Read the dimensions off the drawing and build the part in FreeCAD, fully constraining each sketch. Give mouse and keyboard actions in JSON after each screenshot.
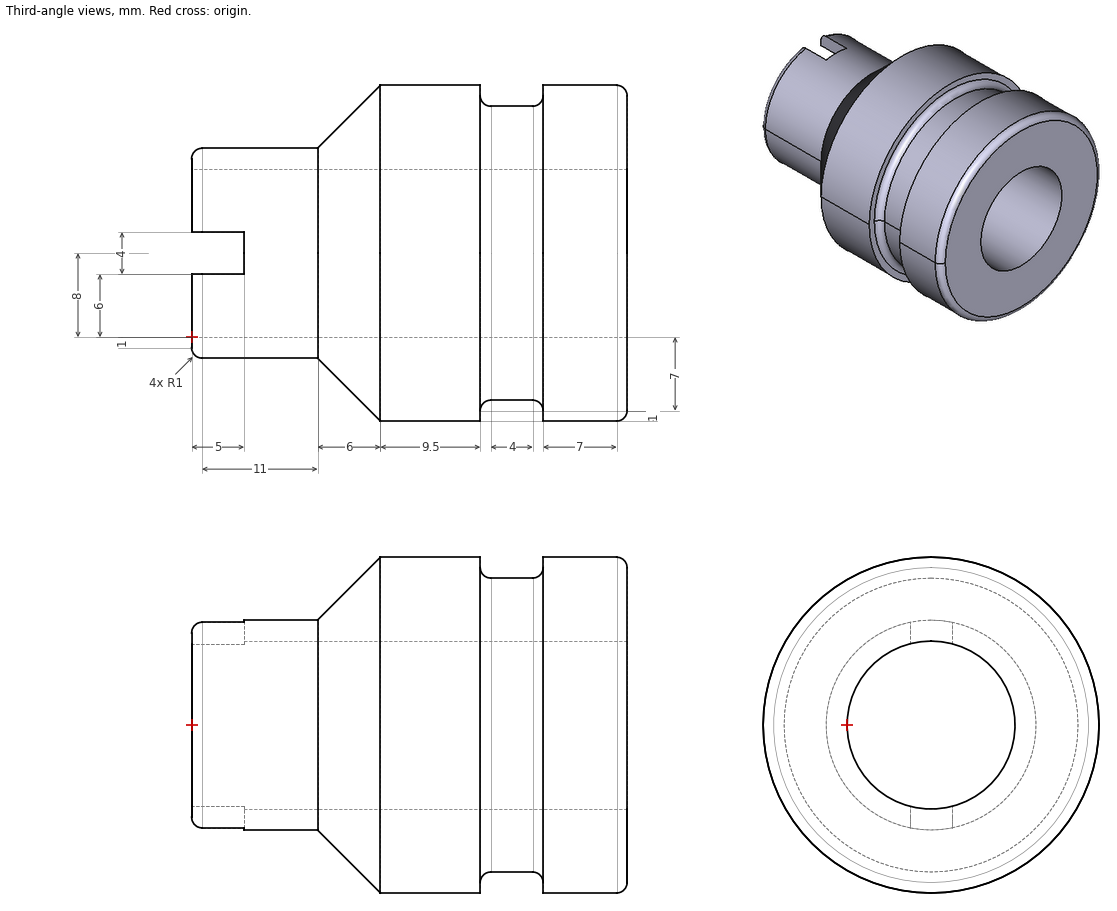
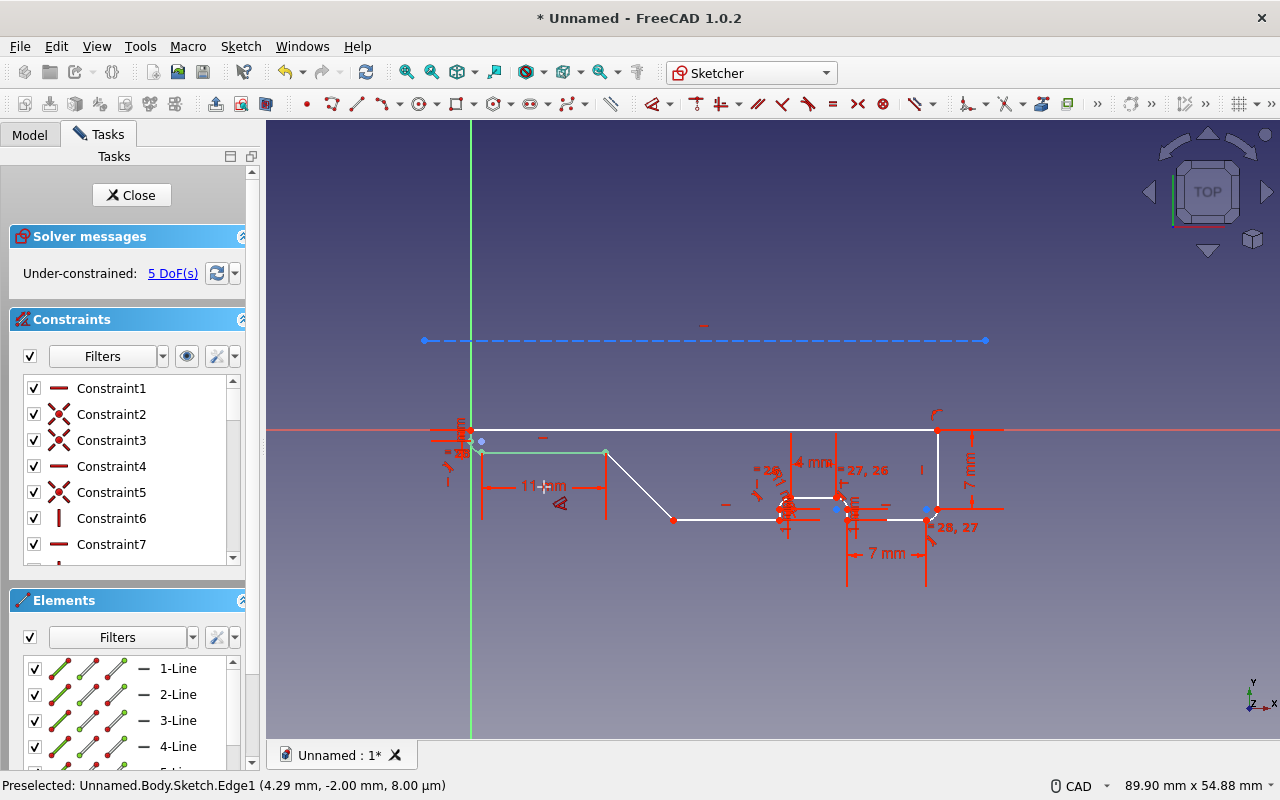
{"action": "left_click", "coordinate": [424, 341]}
{"action": "left_click", "coordinate": [390, 385]}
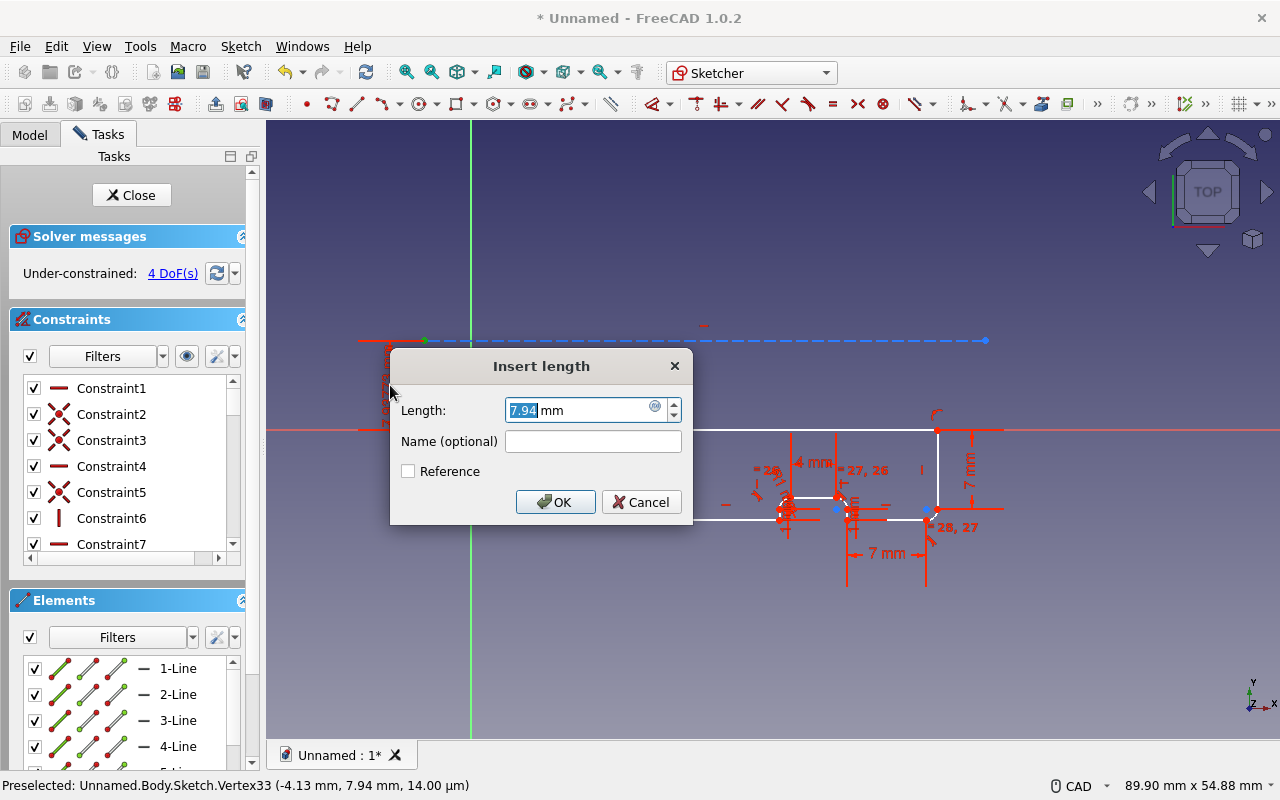
{"action": "type", "text": "8"}
{"action": "key", "text": "Return"}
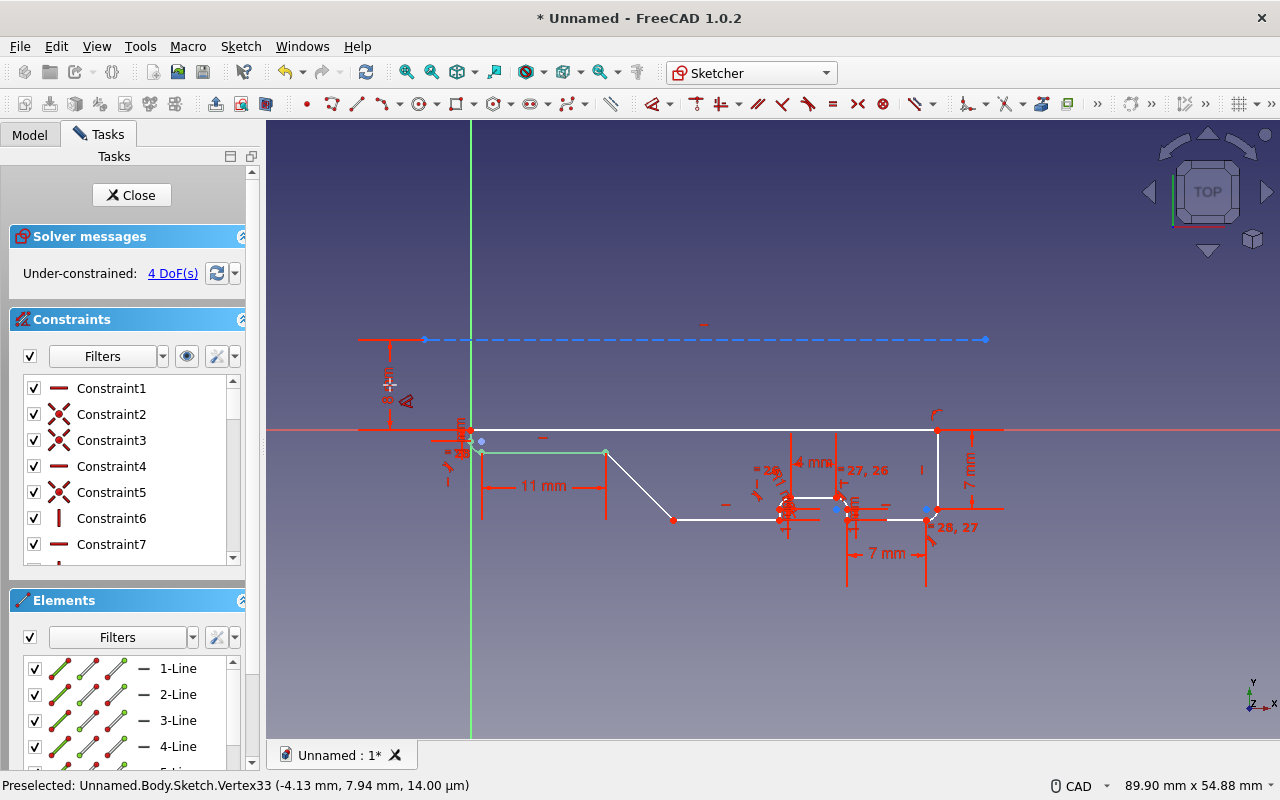
{"action": "left_click", "coordinate": [626, 473]}
{"action": "left_click", "coordinate": [640, 554]}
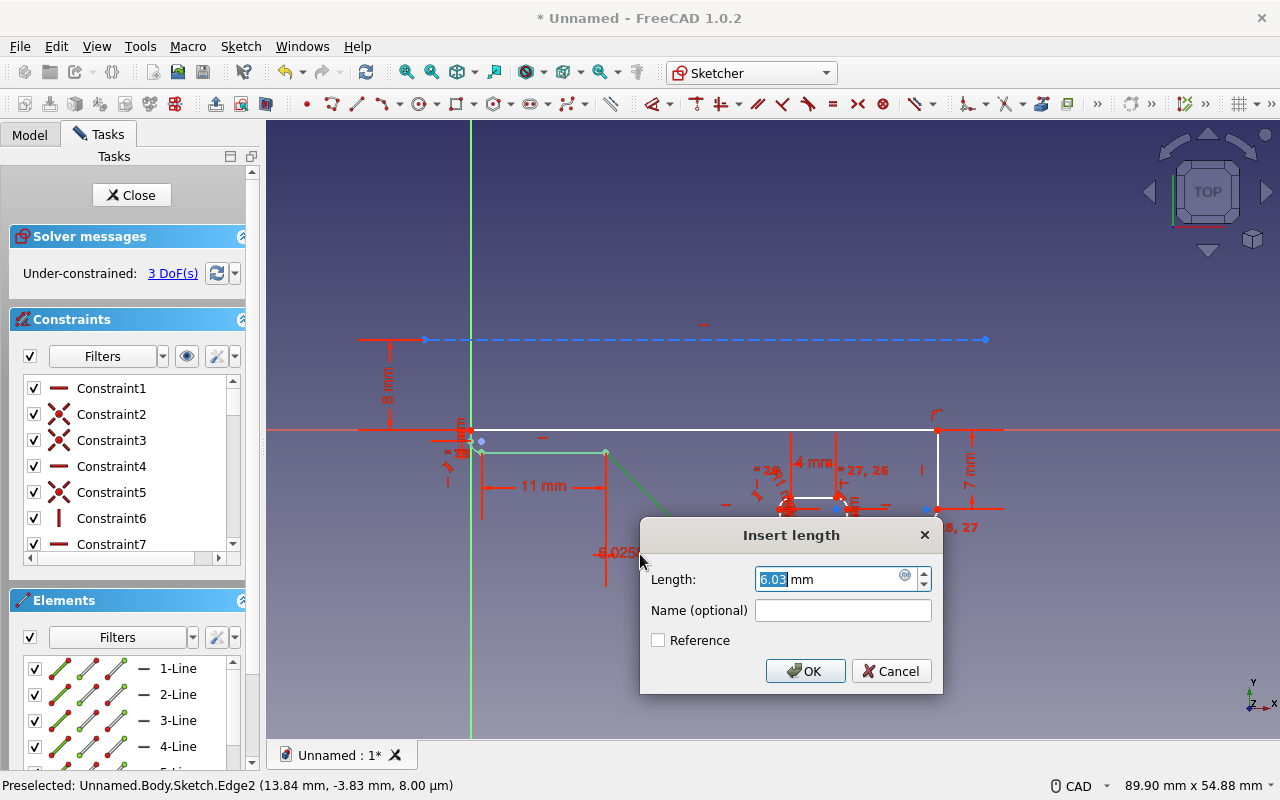
{"action": "type", "text": "6"}
{"action": "key", "text": "Return"}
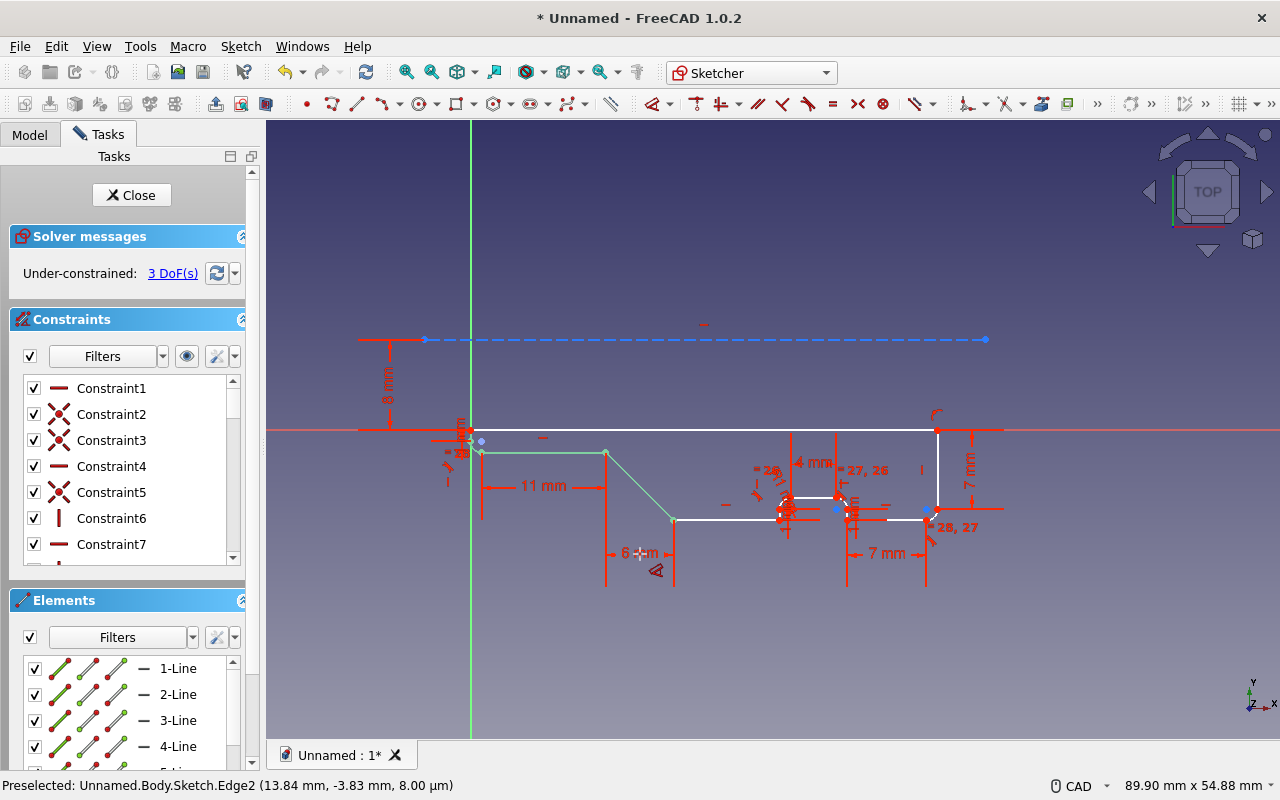
{"action": "left_click", "coordinate": [705, 520]}
{"action": "left_click", "coordinate": [727, 554]}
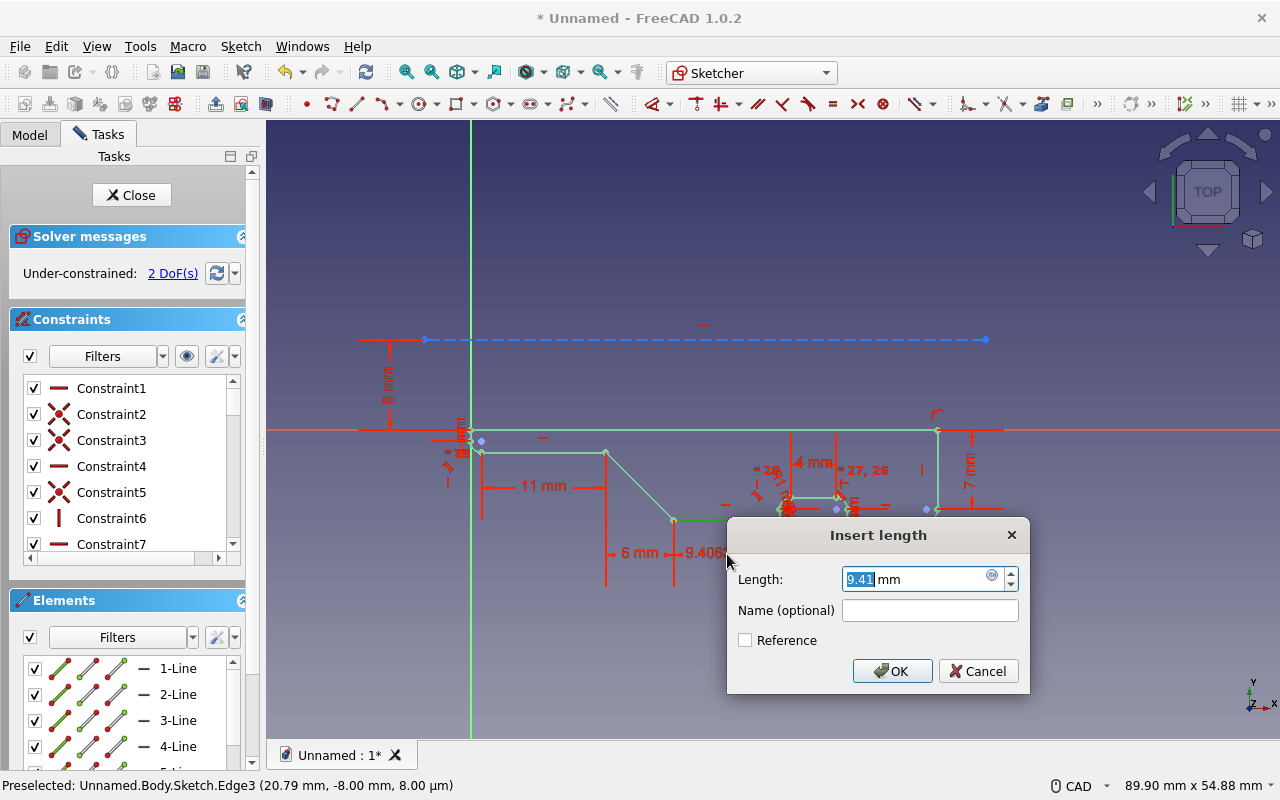
{"action": "type", "text": "9.5"}
{"action": "key", "text": "Return"}
{"action": "key", "text": "Escape"}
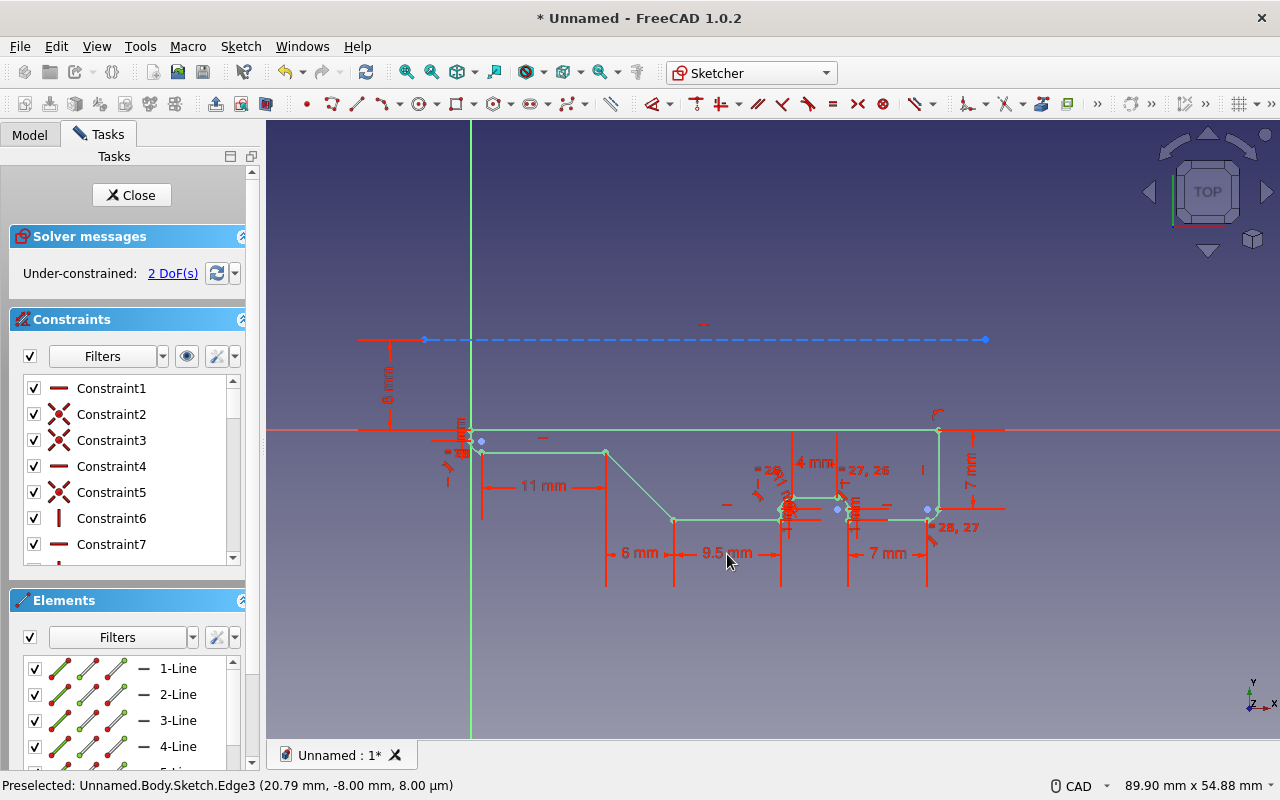
{"action": "left_click", "coordinate": [132, 195]}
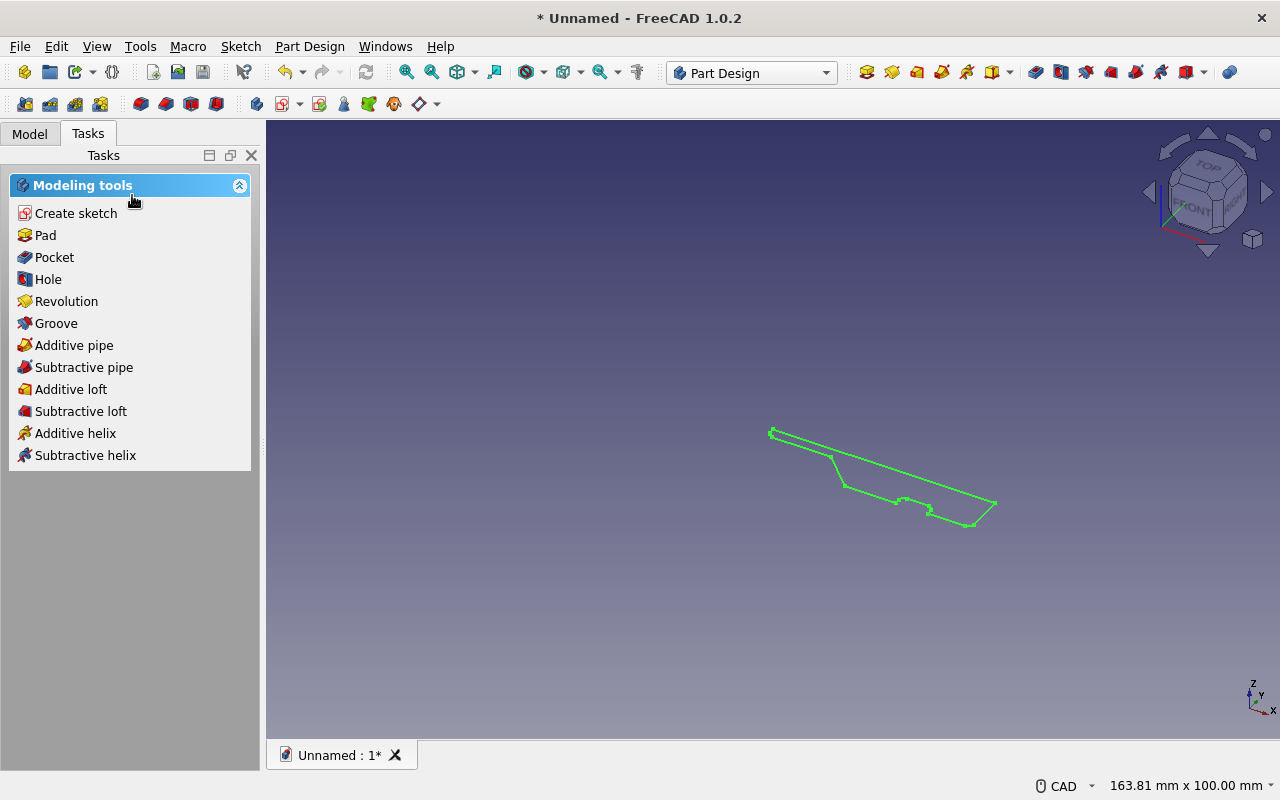
{"action": "left_click", "coordinate": [892, 72]}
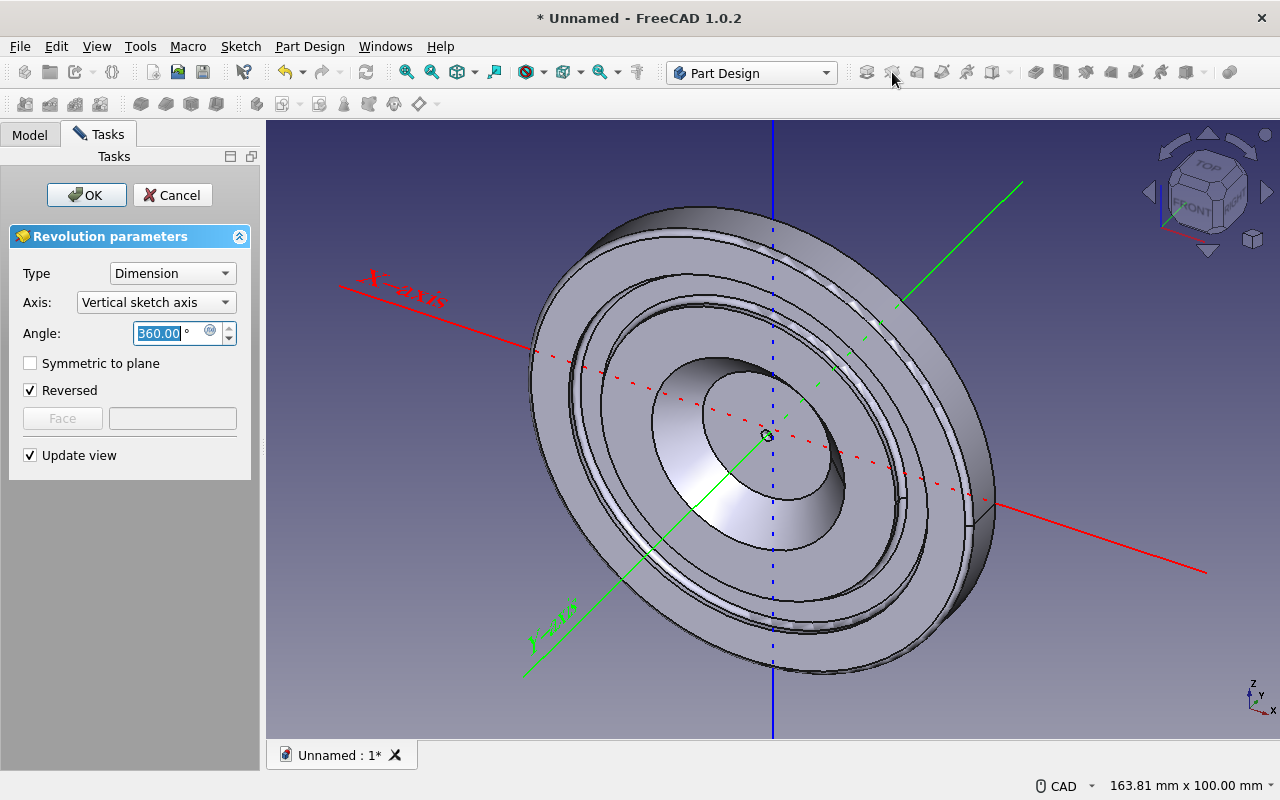
{"action": "left_click", "coordinate": [157, 302]}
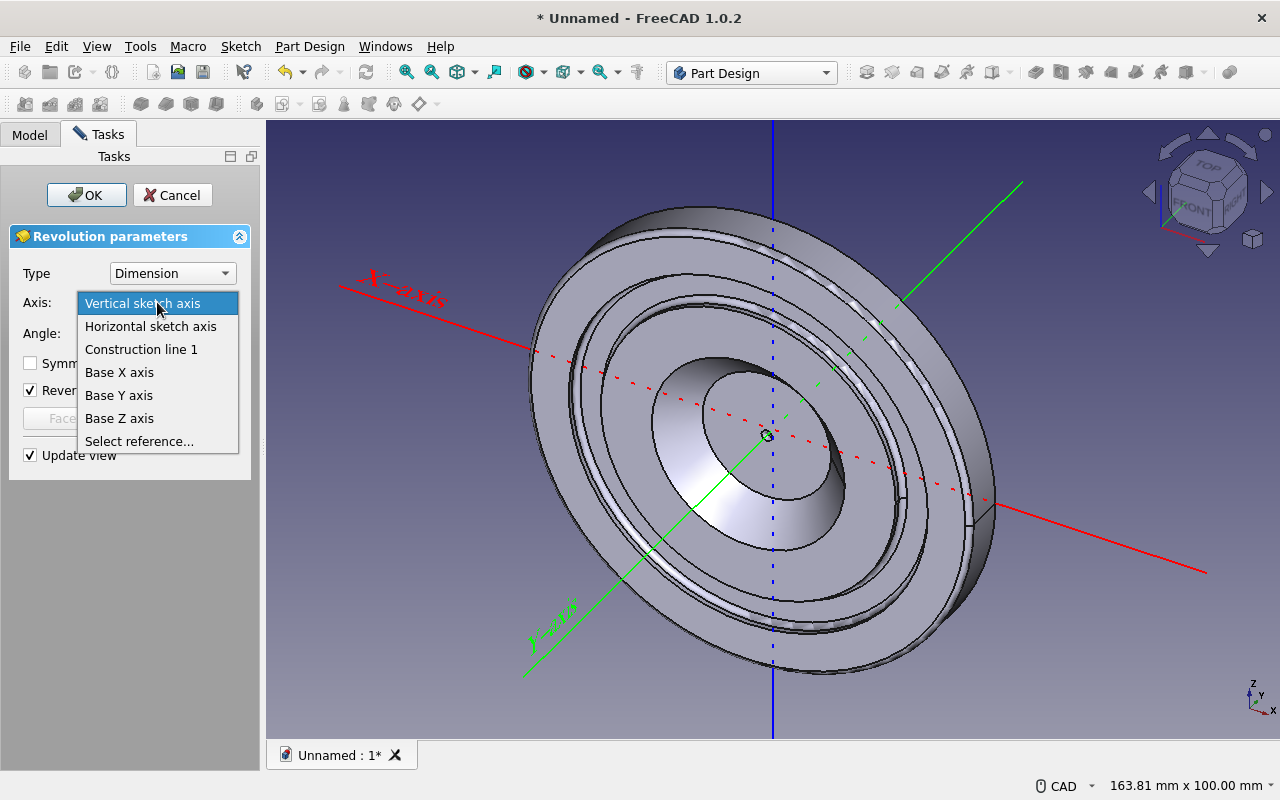
{"action": "left_click", "coordinate": [156, 350]}